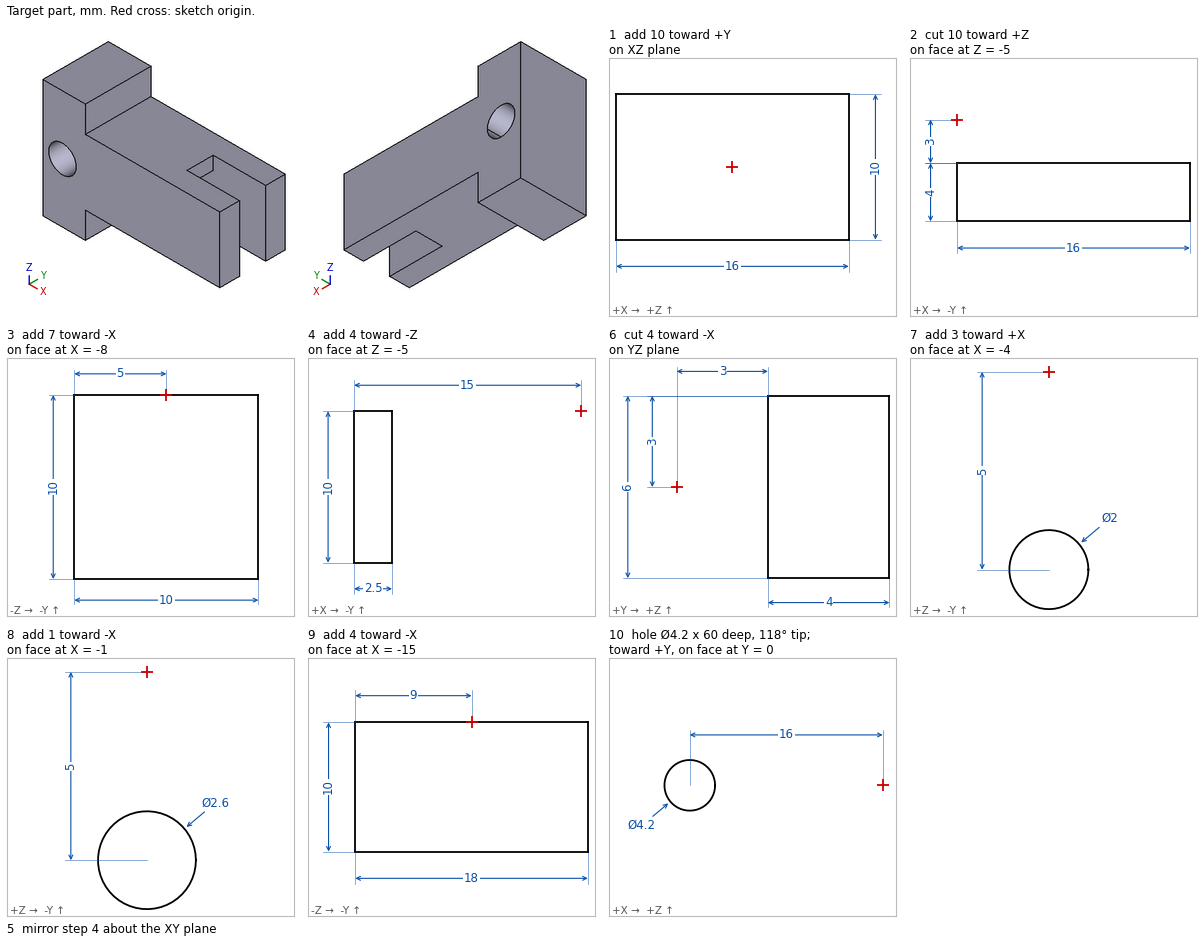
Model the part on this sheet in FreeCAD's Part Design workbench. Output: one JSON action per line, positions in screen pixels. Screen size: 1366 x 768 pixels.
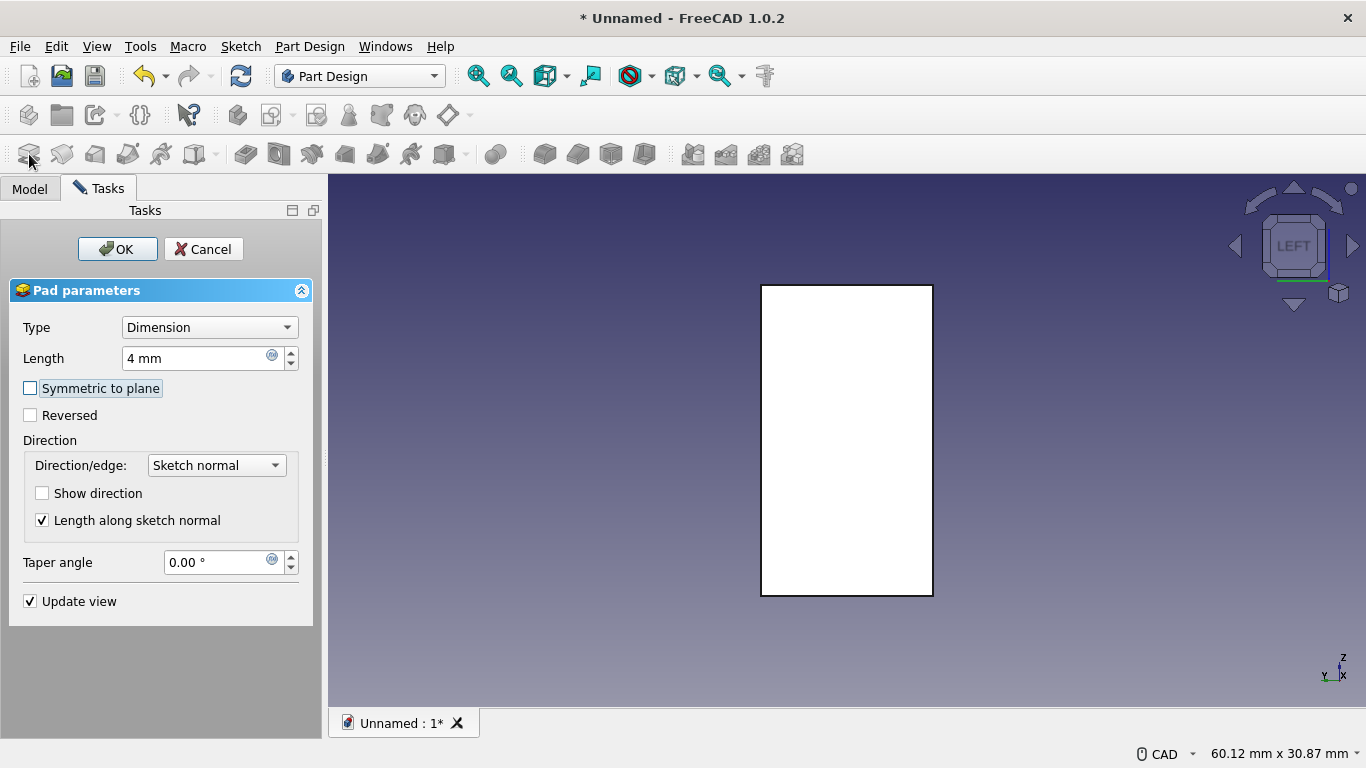
{"action": "left_click", "coordinate": [118, 249]}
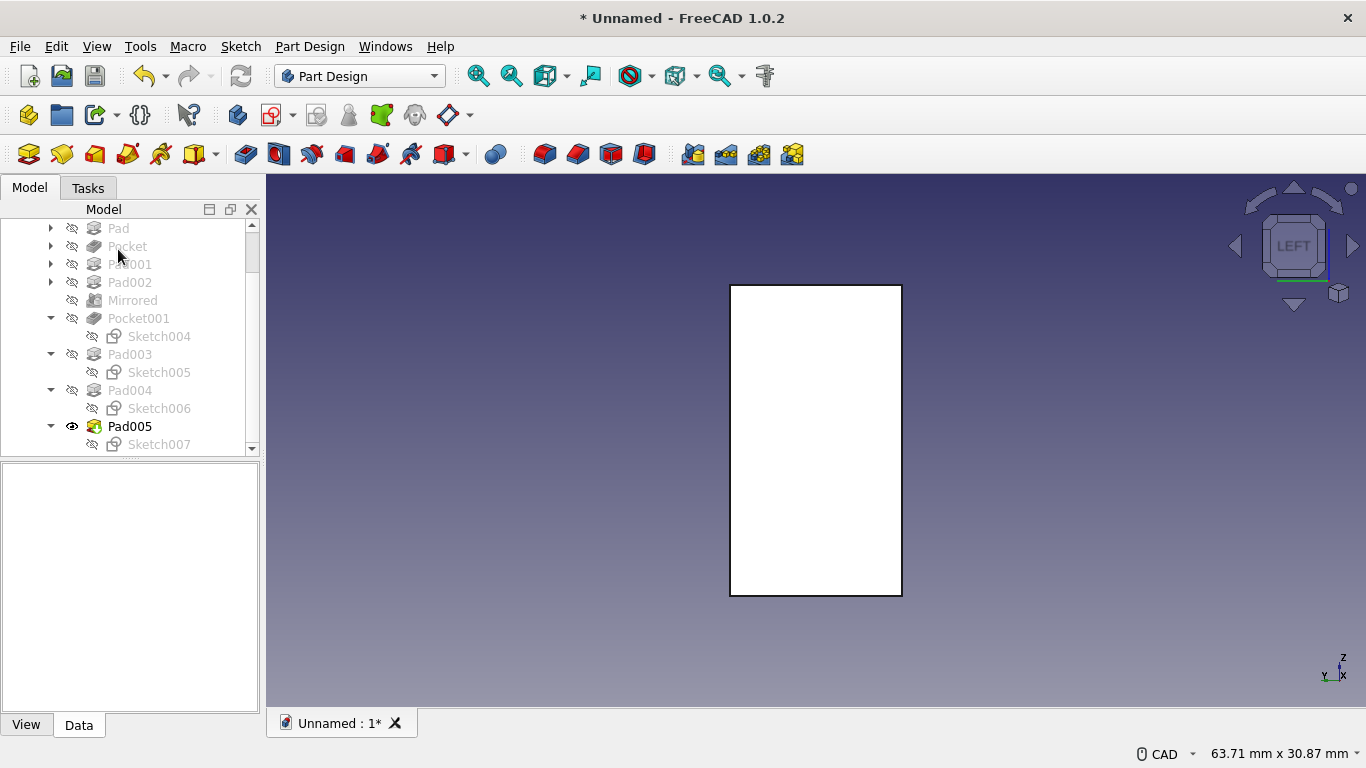
{"action": "key", "text": "0"}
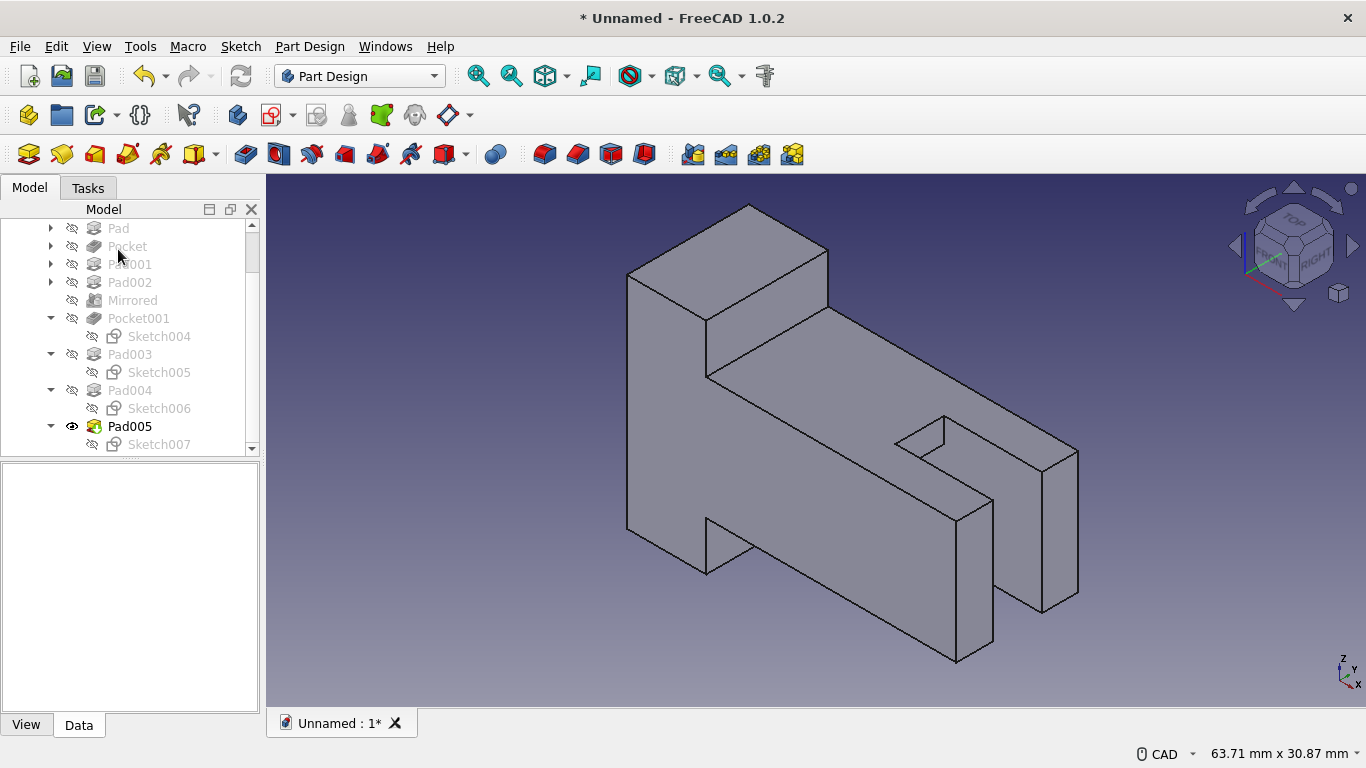
{"action": "left_click", "coordinate": [479, 76]}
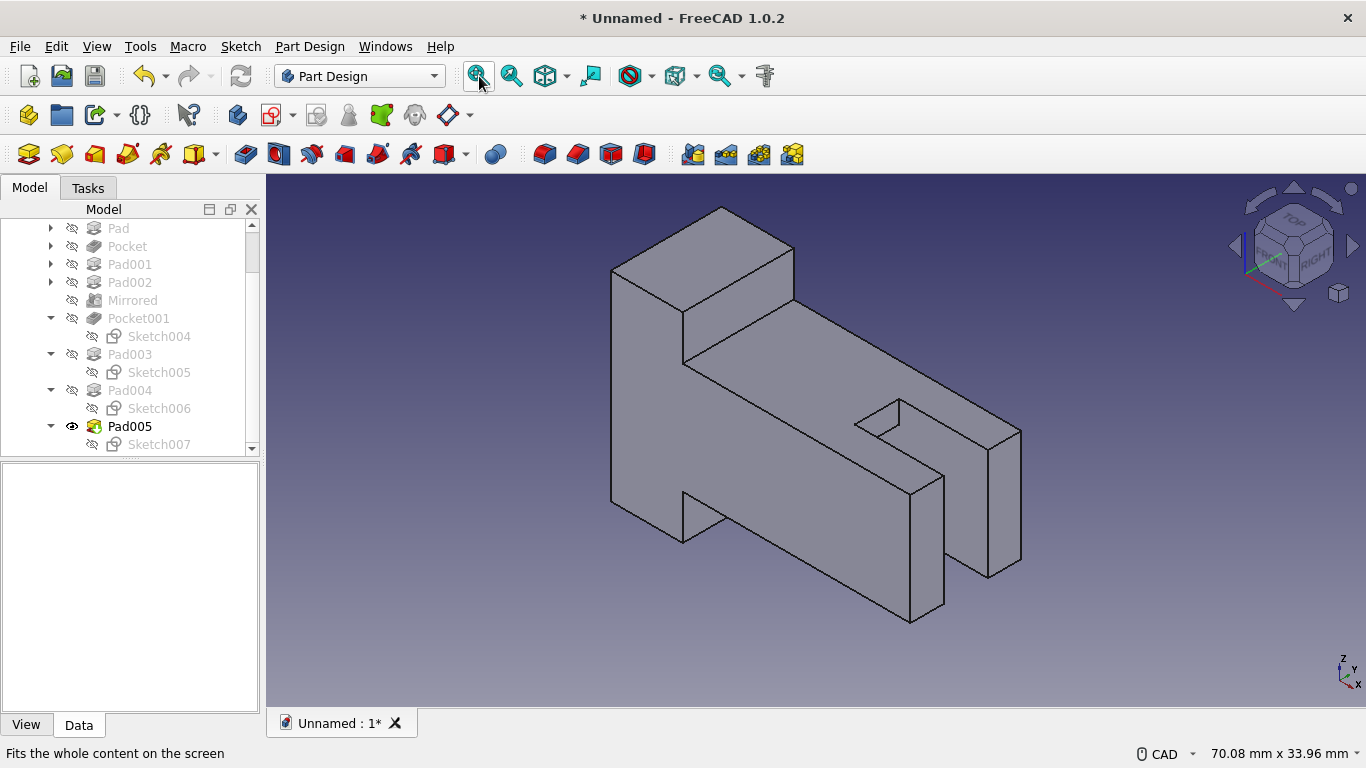
{"action": "left_click", "coordinate": [675, 422]}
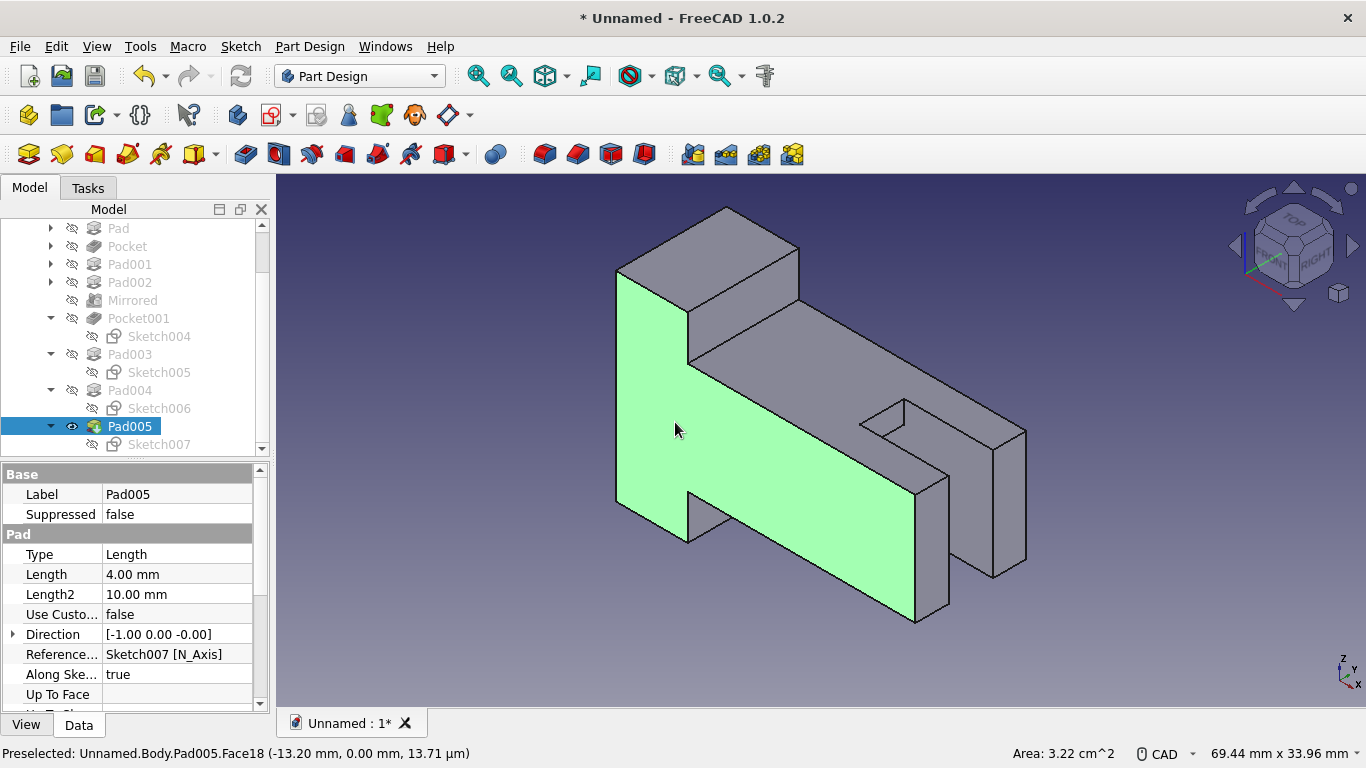
{"action": "left_click", "coordinate": [270, 116]}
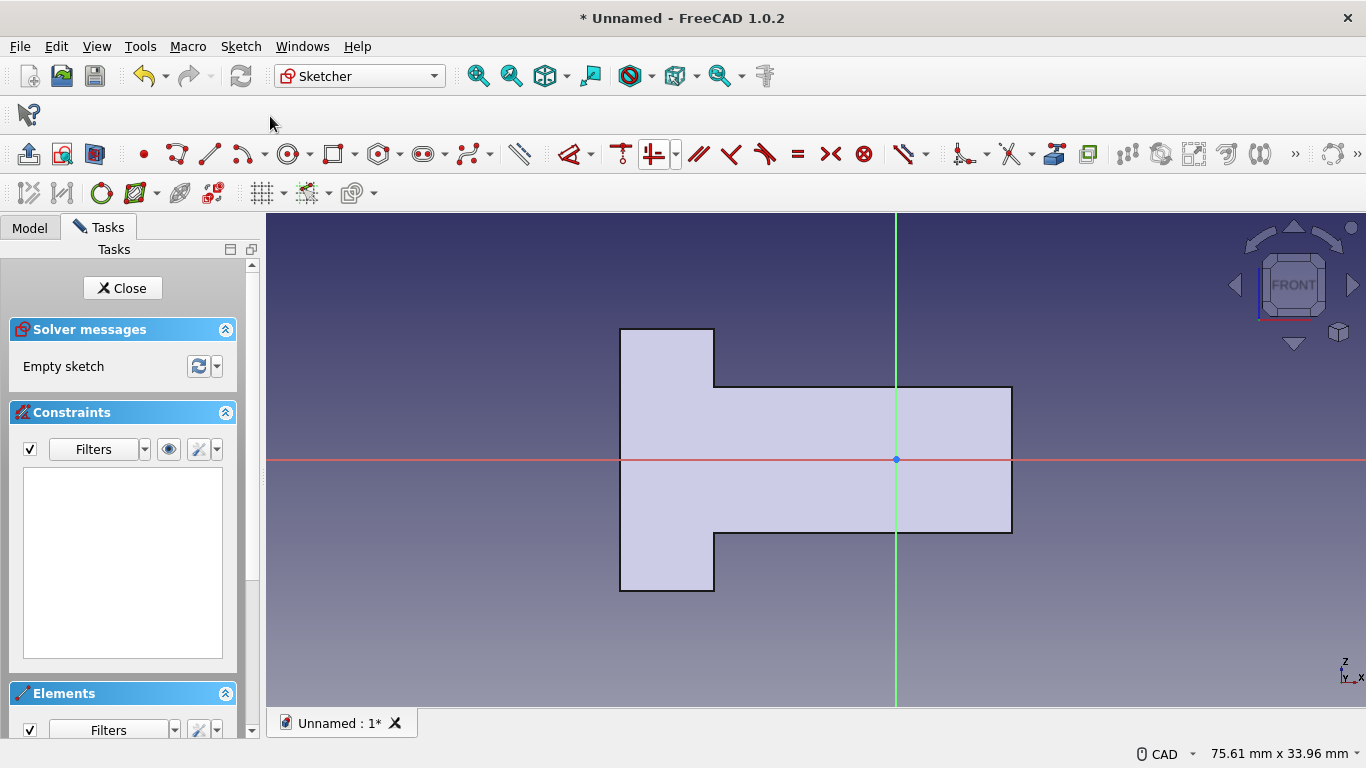
{"action": "scroll", "coordinate": [642, 460], "scroll_direction": "up", "scroll_amount": 8}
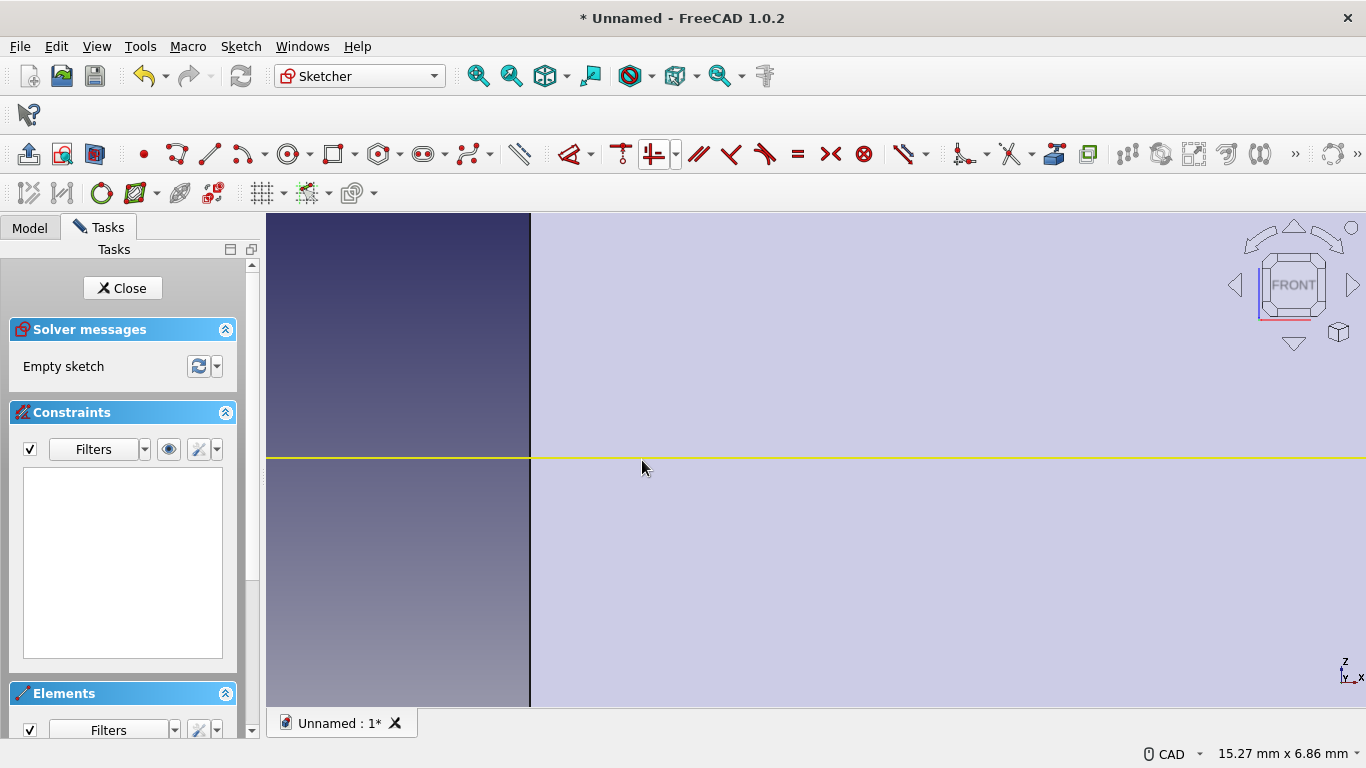
{"action": "left_click", "coordinate": [288, 154]}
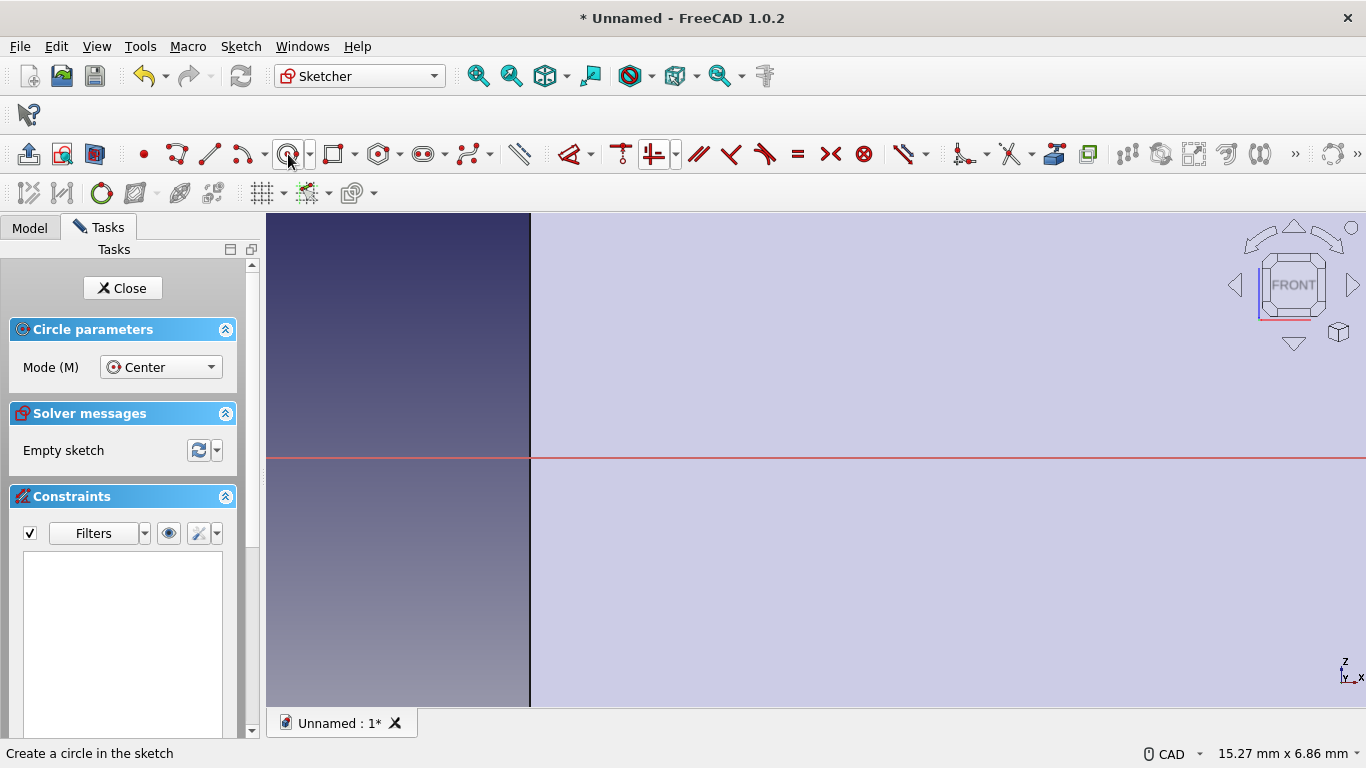
{"action": "left_click", "coordinate": [746, 458]}
{"action": "left_click", "coordinate": [853, 351]}
{"action": "key", "text": "Escape"}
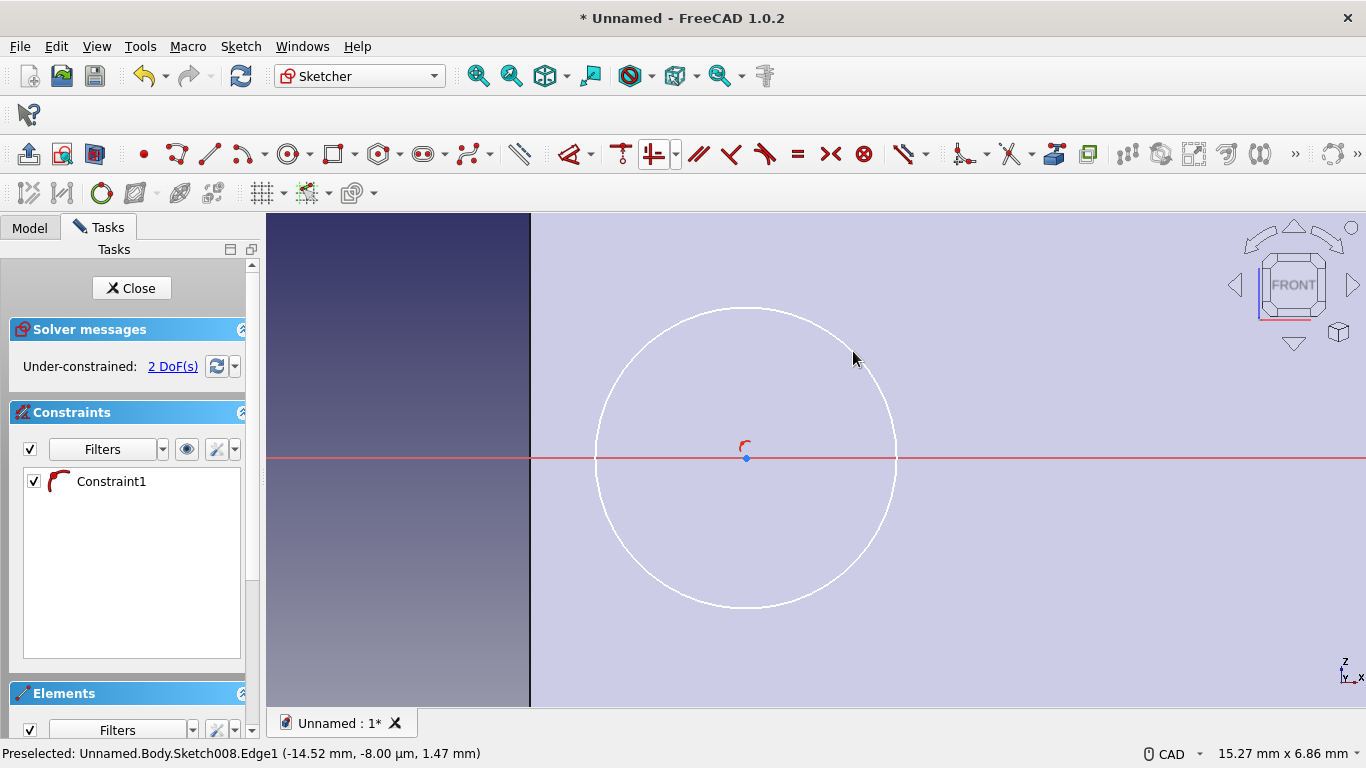
{"action": "left_click", "coordinate": [568, 154]}